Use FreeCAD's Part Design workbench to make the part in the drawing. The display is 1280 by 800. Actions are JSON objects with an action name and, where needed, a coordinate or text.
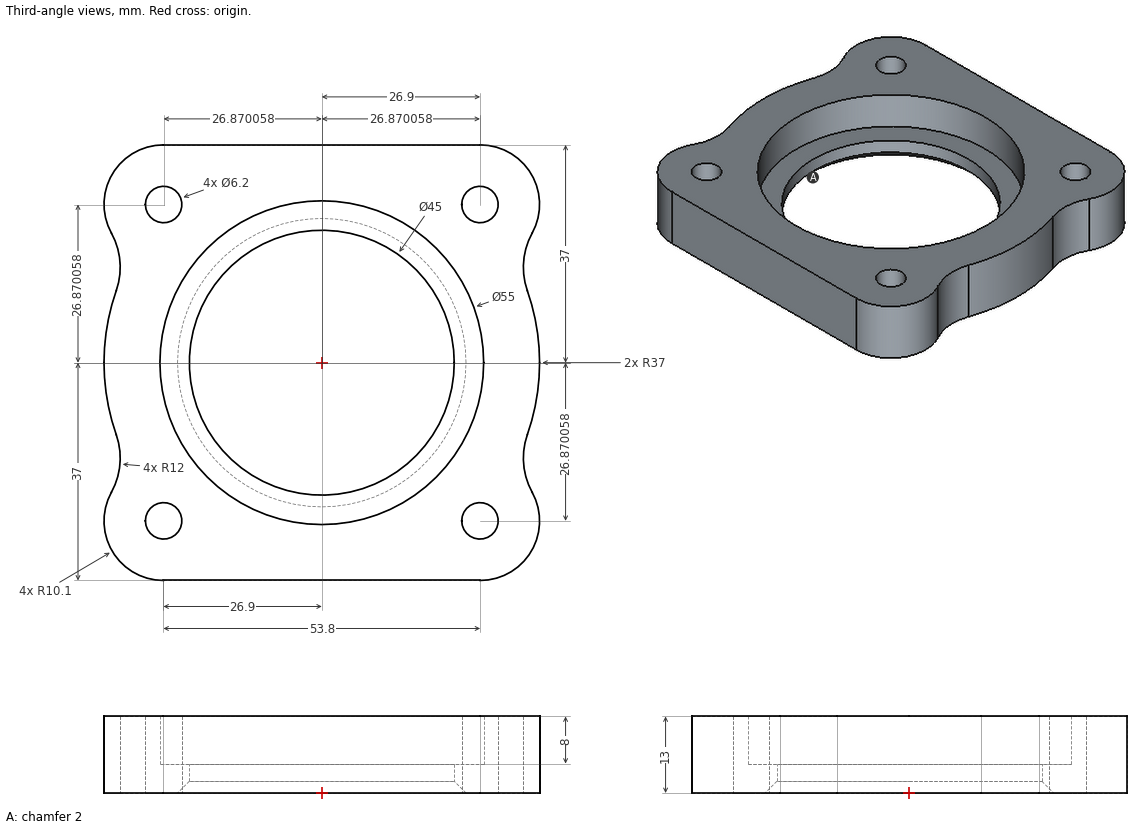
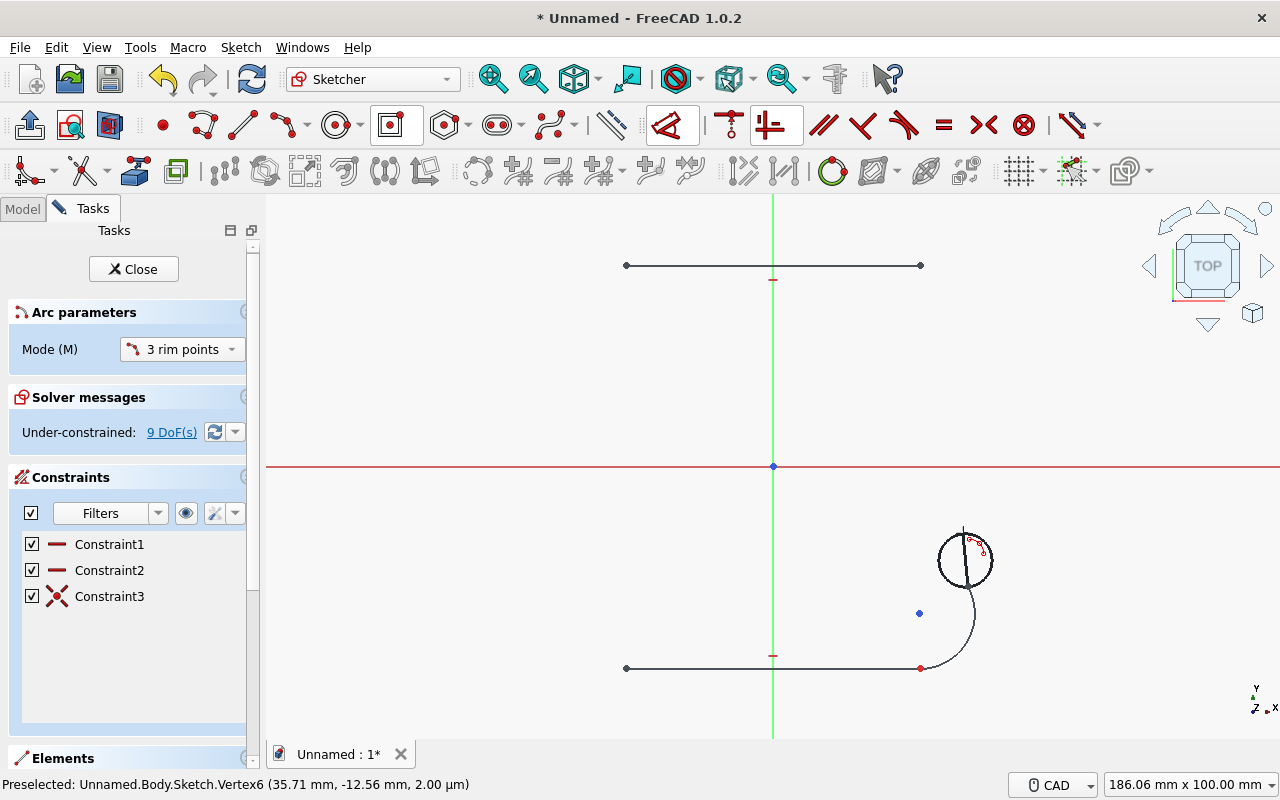
{"action": "scroll", "coordinate": [960, 560], "scroll_direction": "up", "scroll_amount": 6}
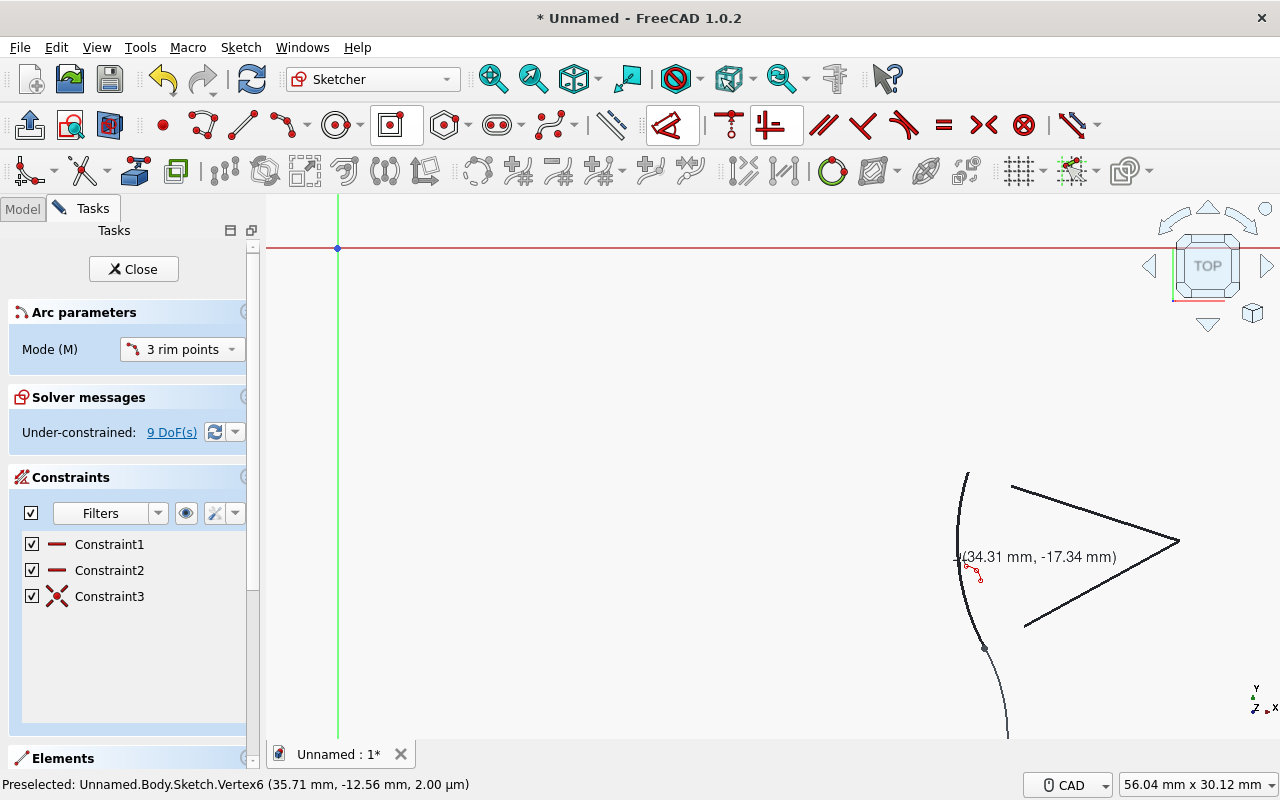
{"action": "left_click", "coordinate": [958, 559]}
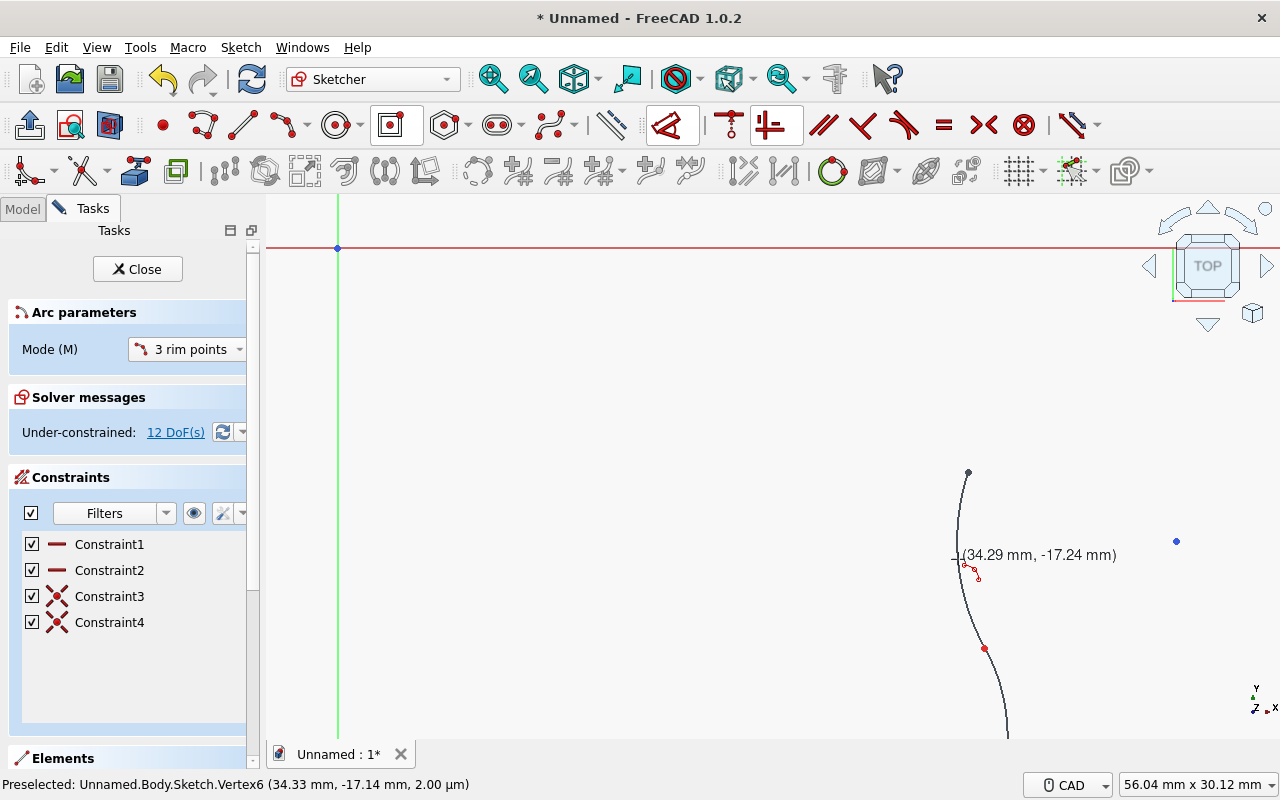
{"action": "left_click", "coordinate": [968, 472]}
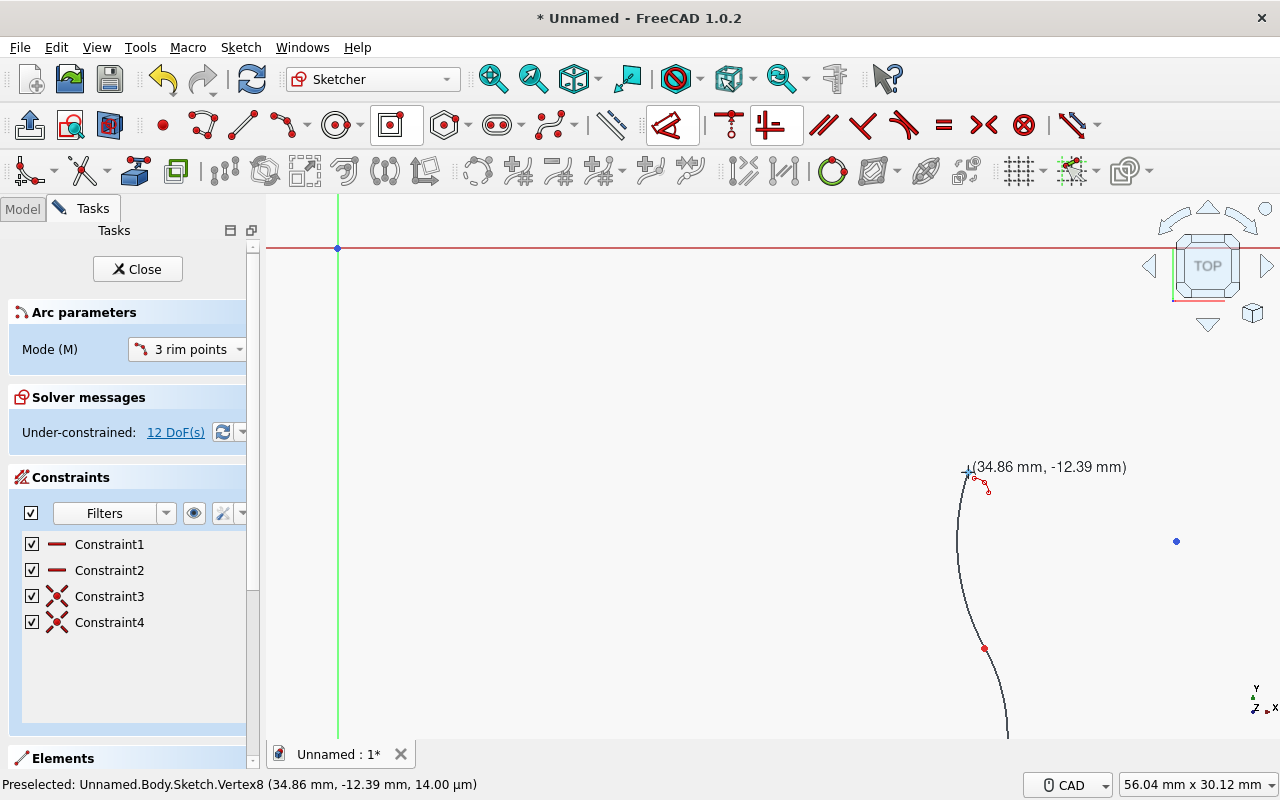
{"action": "scroll", "coordinate": [825, 538], "scroll_direction": "down", "scroll_amount": 7}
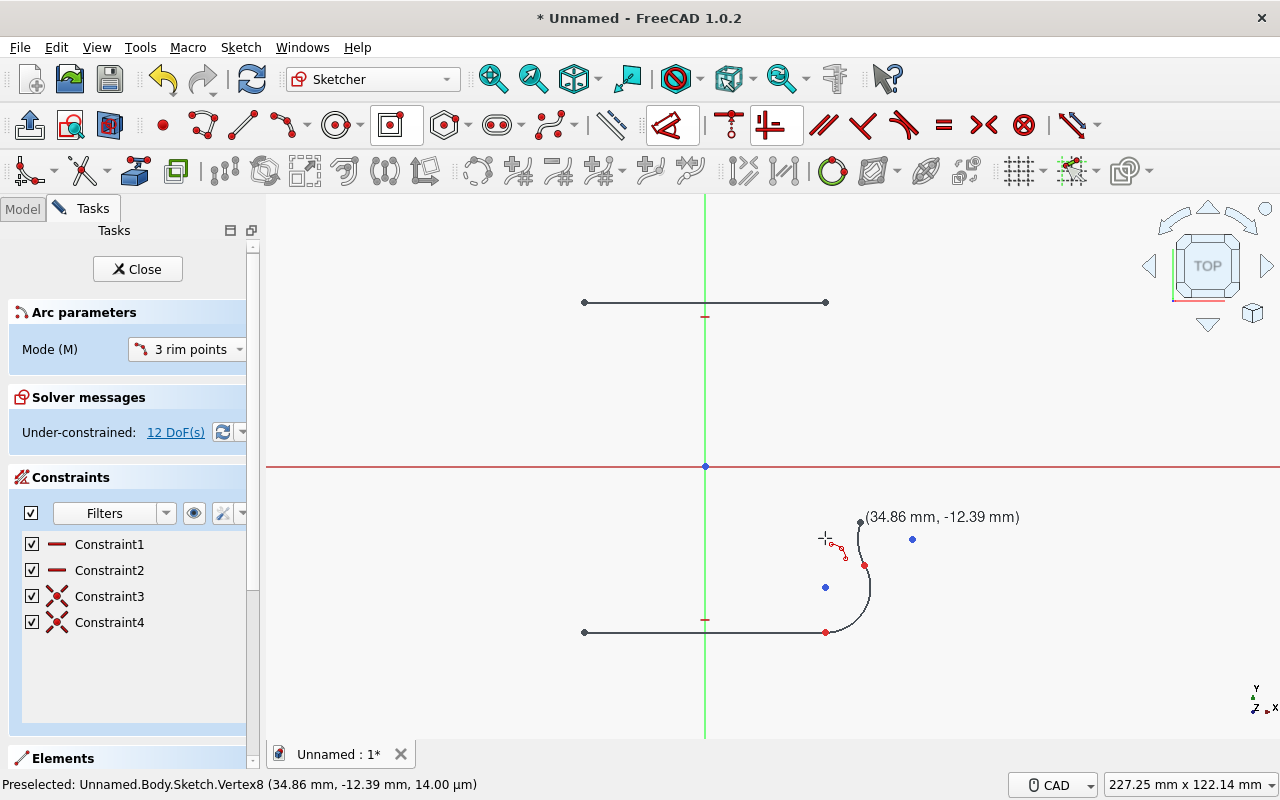
{"action": "left_click", "coordinate": [861, 412]}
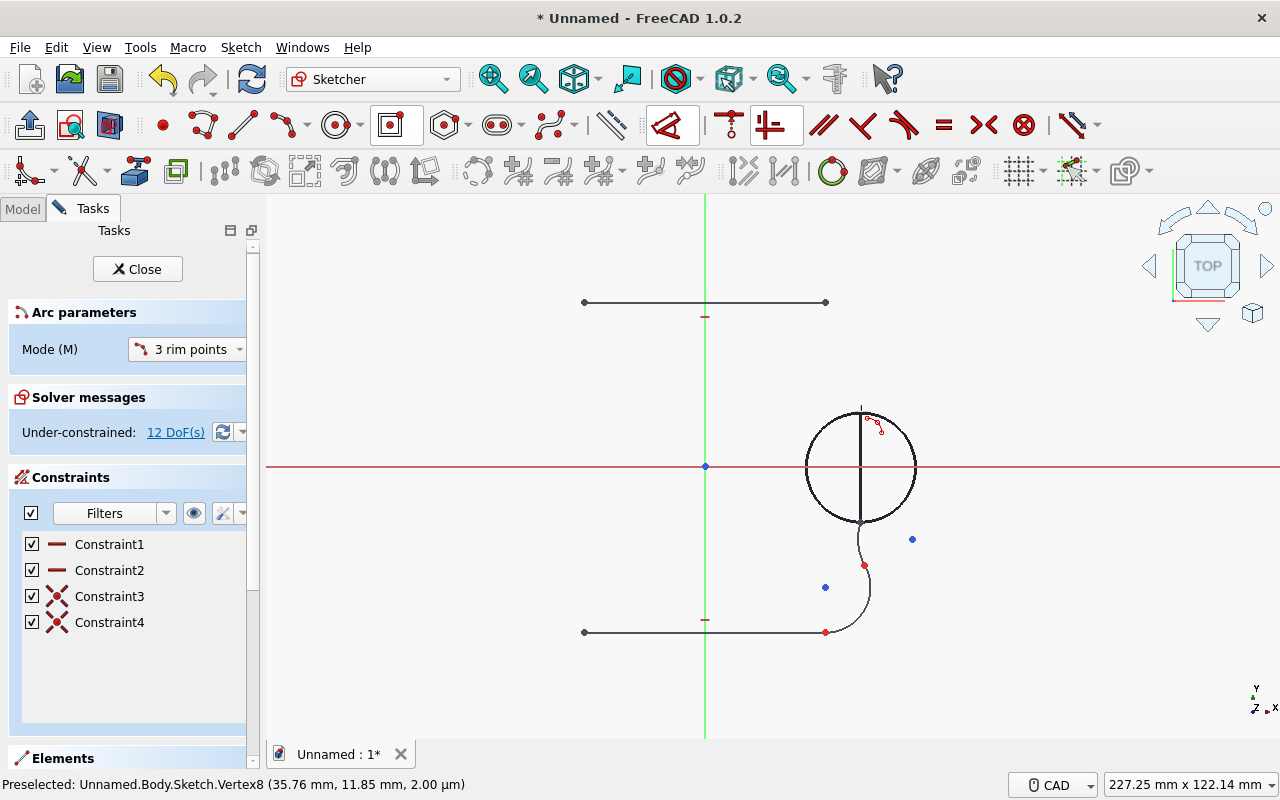
{"action": "scroll", "coordinate": [870, 478], "scroll_direction": "up", "scroll_amount": 3}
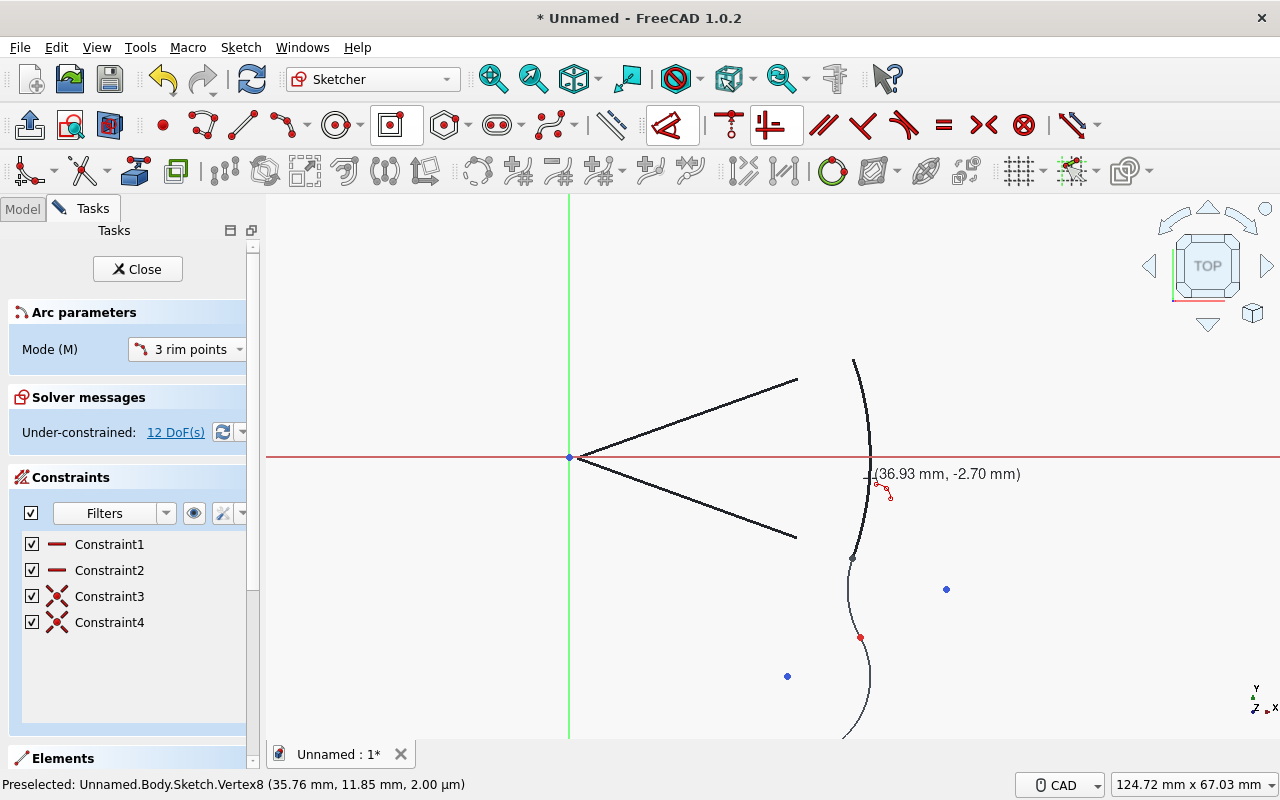
{"action": "left_click", "coordinate": [869, 478]}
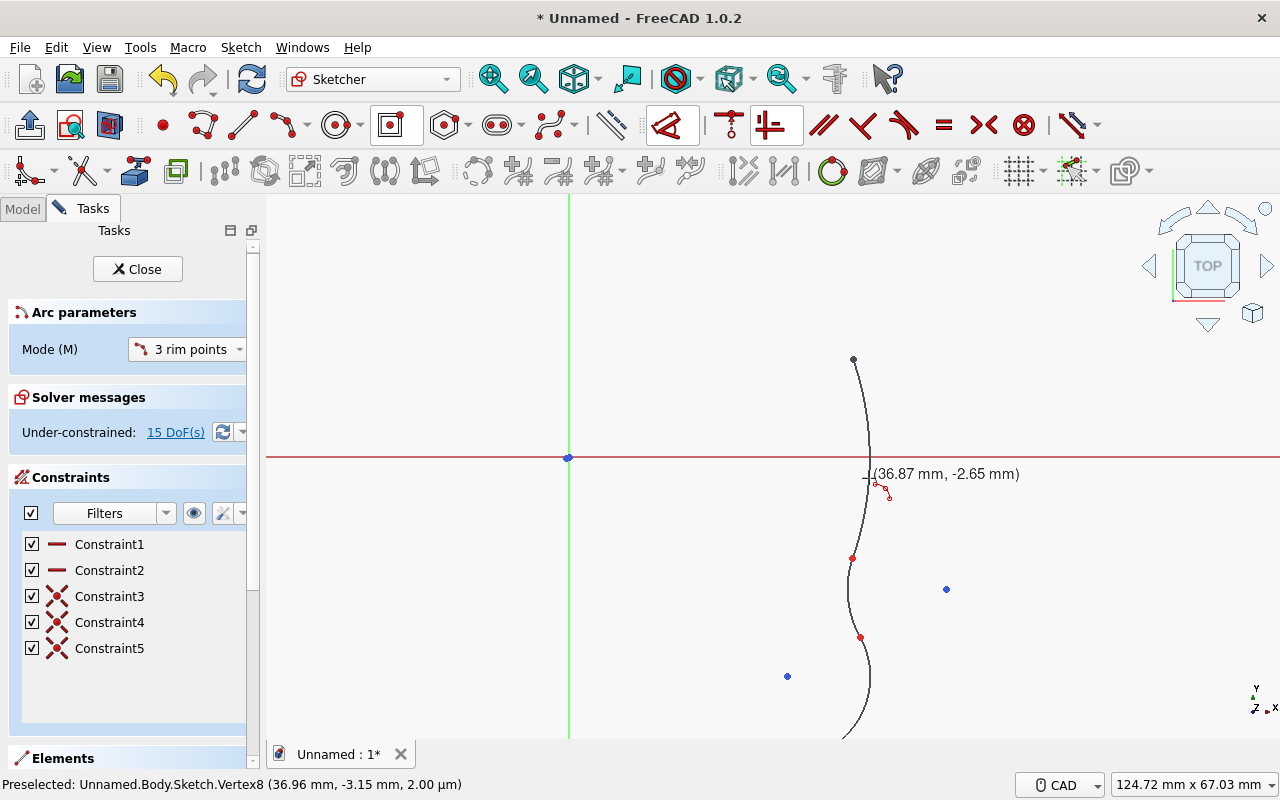
{"action": "left_click", "coordinate": [853, 359]}
{"action": "left_click", "coordinate": [860, 278]}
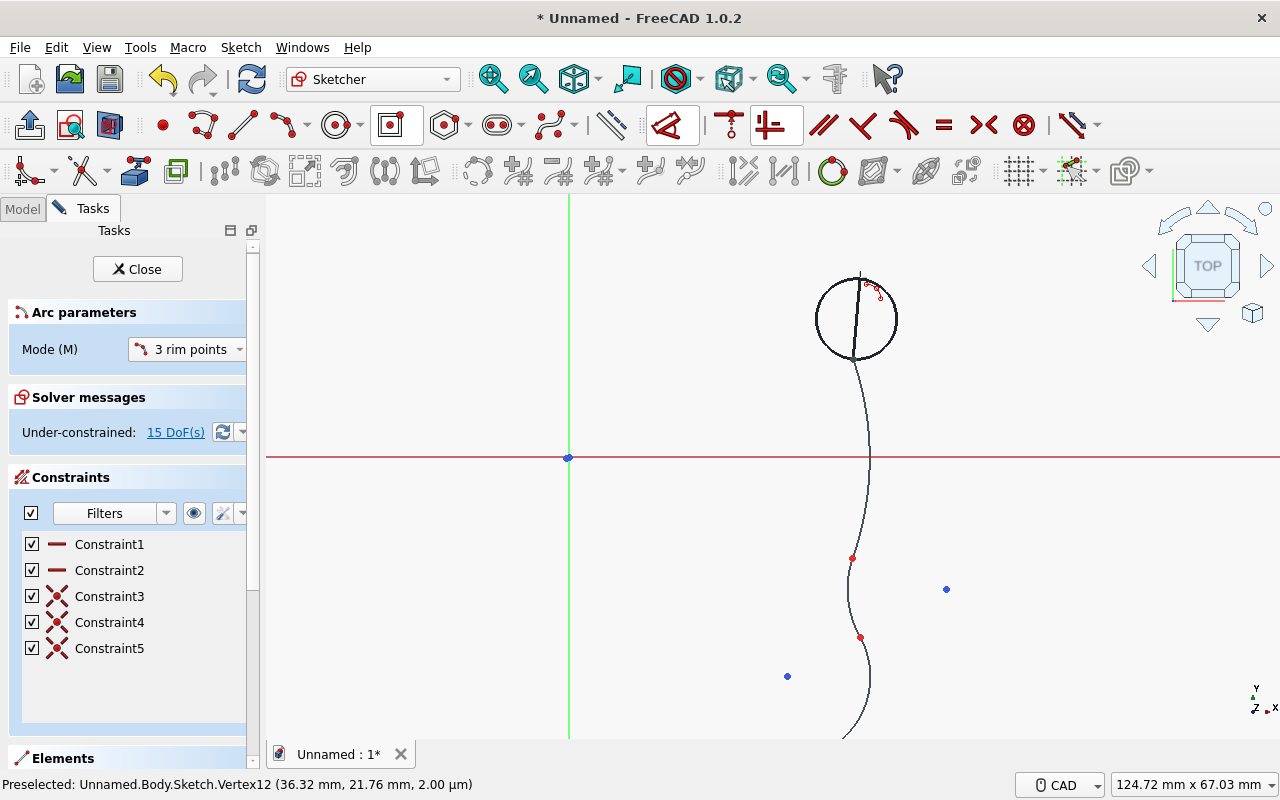
{"action": "scroll", "coordinate": [848, 318], "scroll_direction": "up", "scroll_amount": 4}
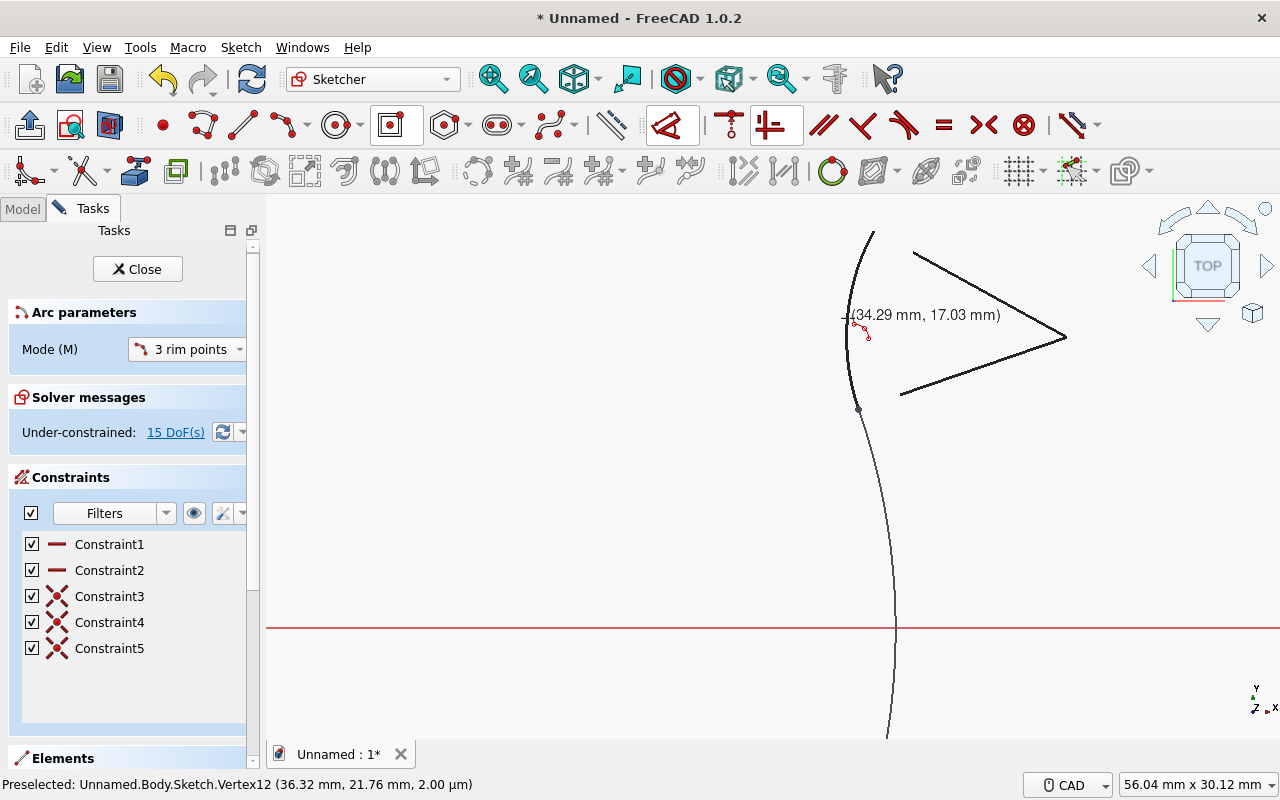
{"action": "left_click", "coordinate": [847, 317]}